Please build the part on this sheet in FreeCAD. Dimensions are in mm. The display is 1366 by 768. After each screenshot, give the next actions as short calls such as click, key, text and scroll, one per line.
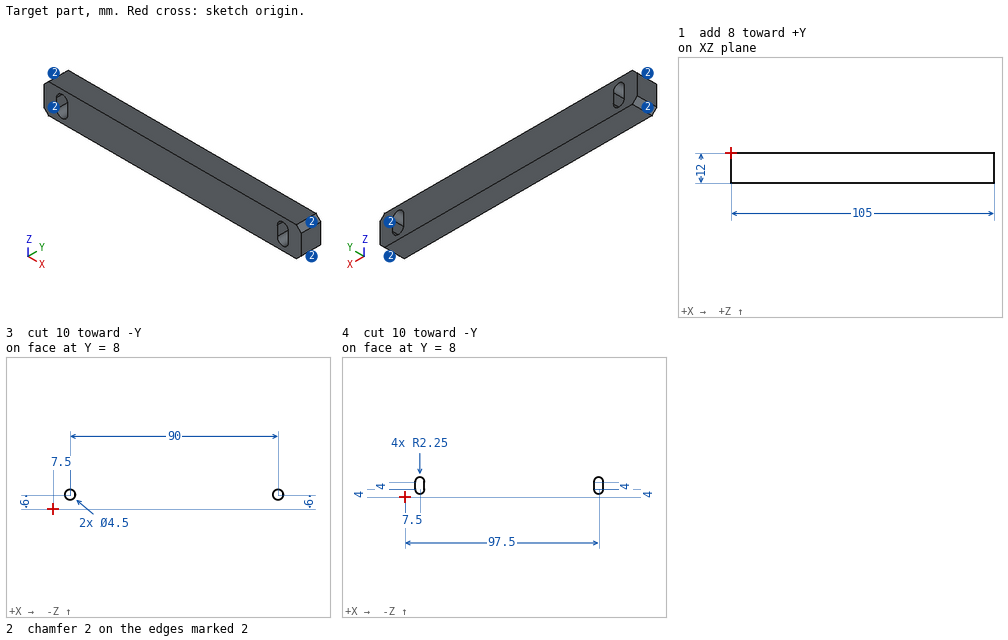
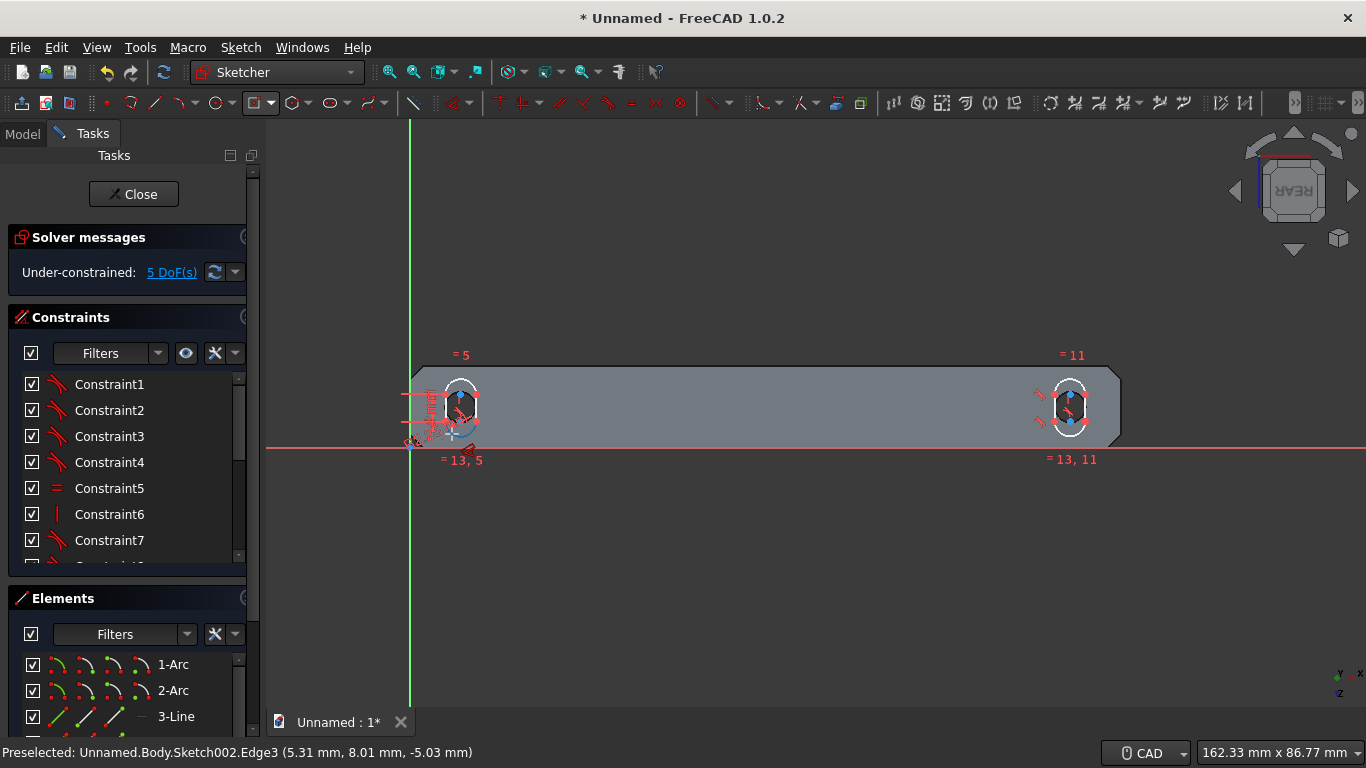
scroll(1055, 413, up, 3)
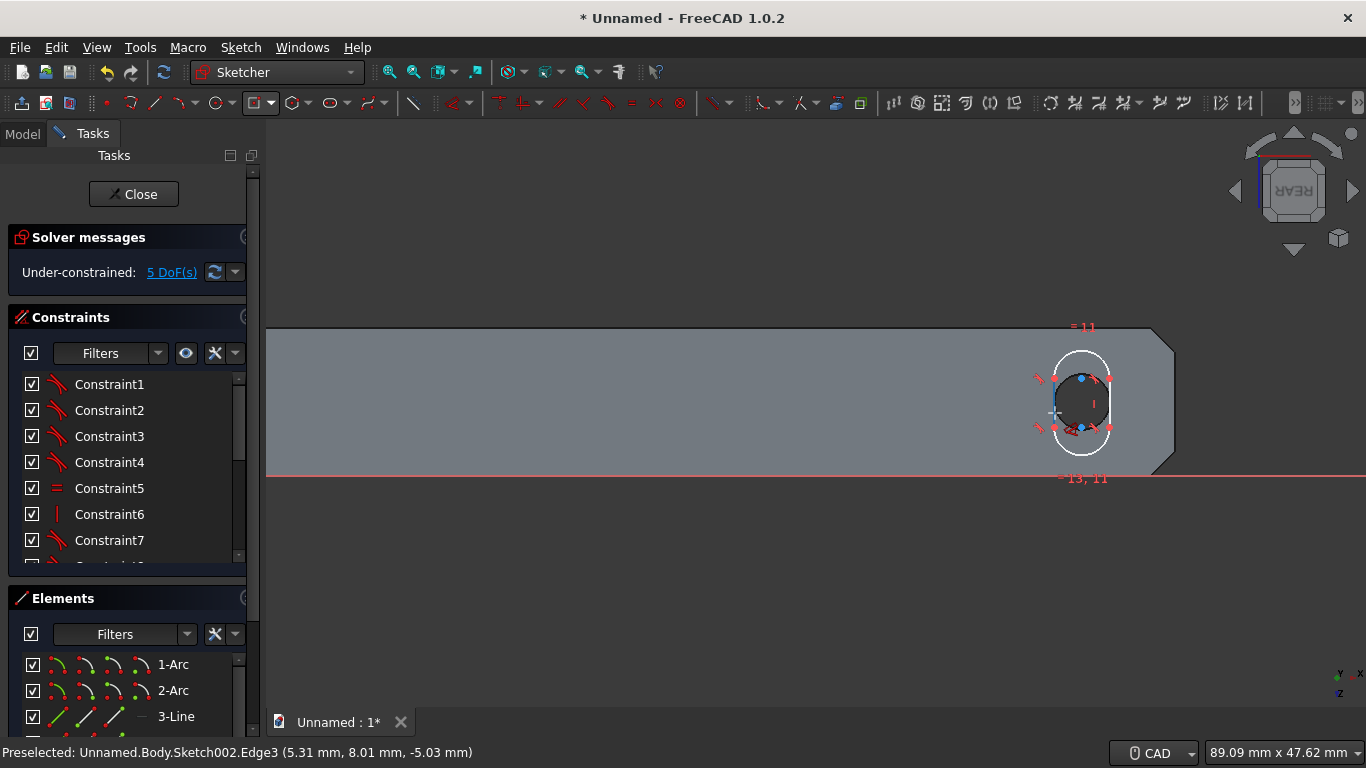
click(1054, 413)
click(1088, 403)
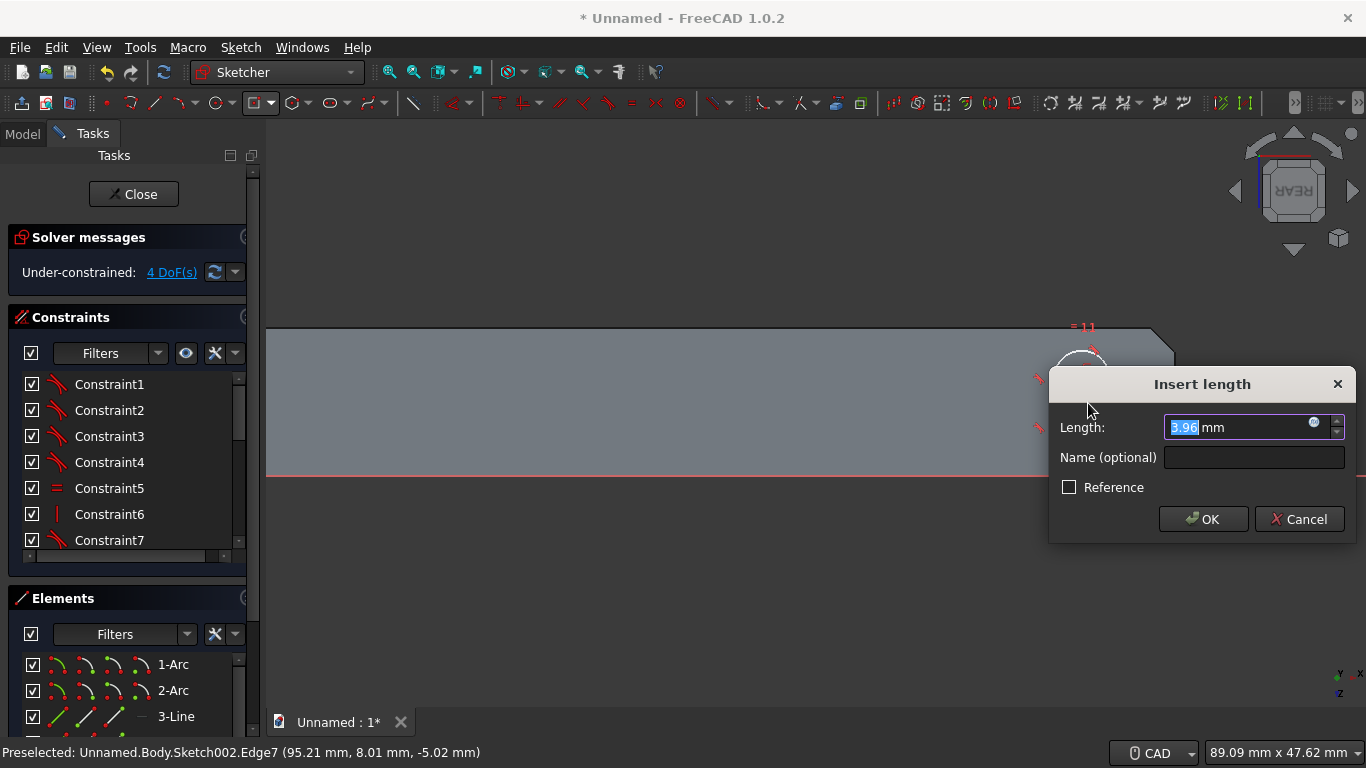
text(4)
key(Return)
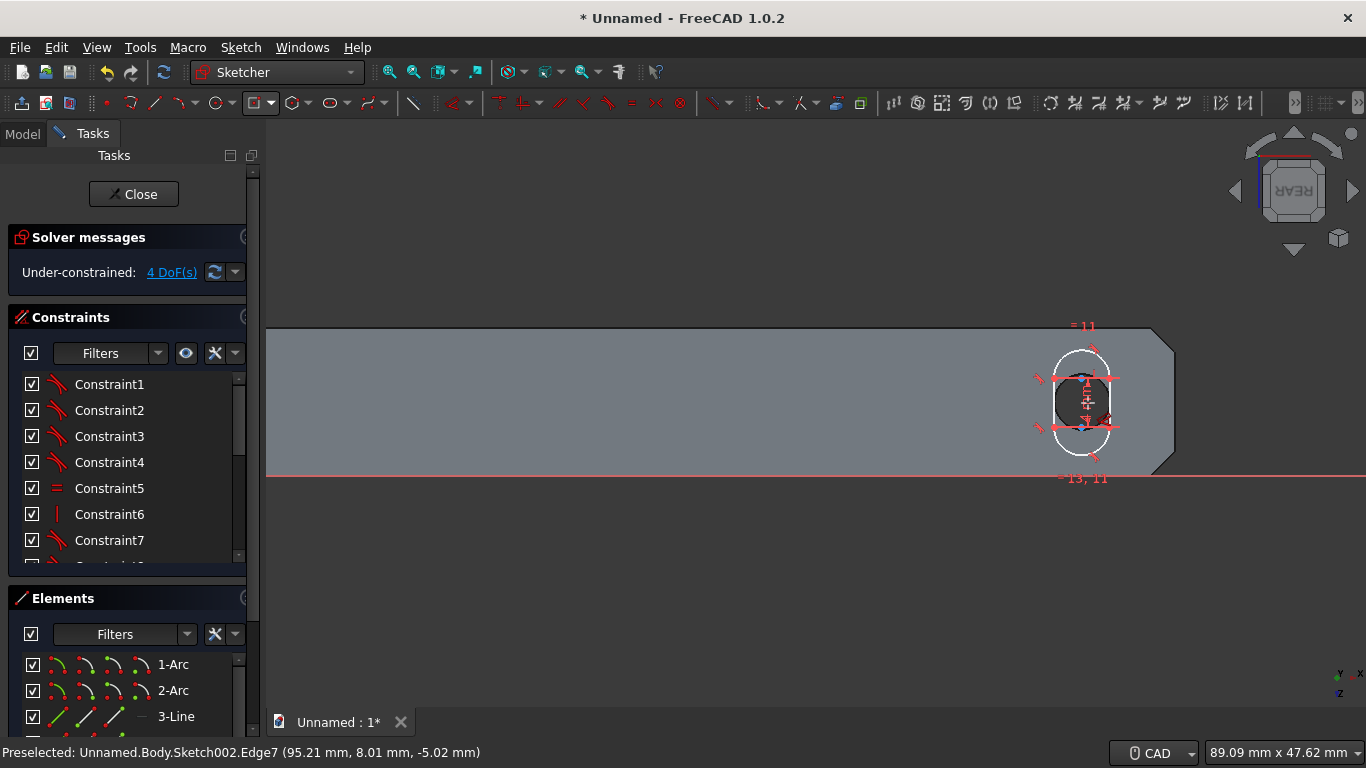
scroll(1056, 413, down, 3)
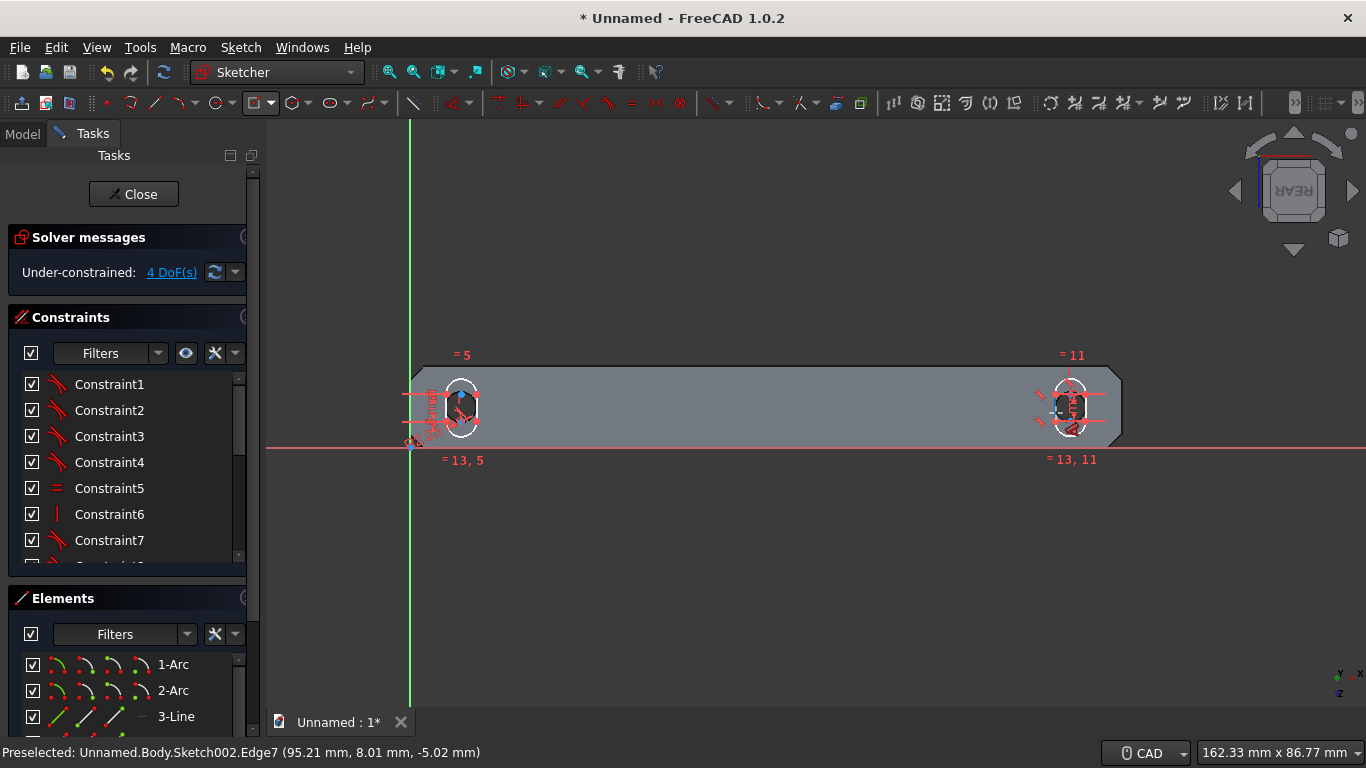
scroll(446, 422, up, 2)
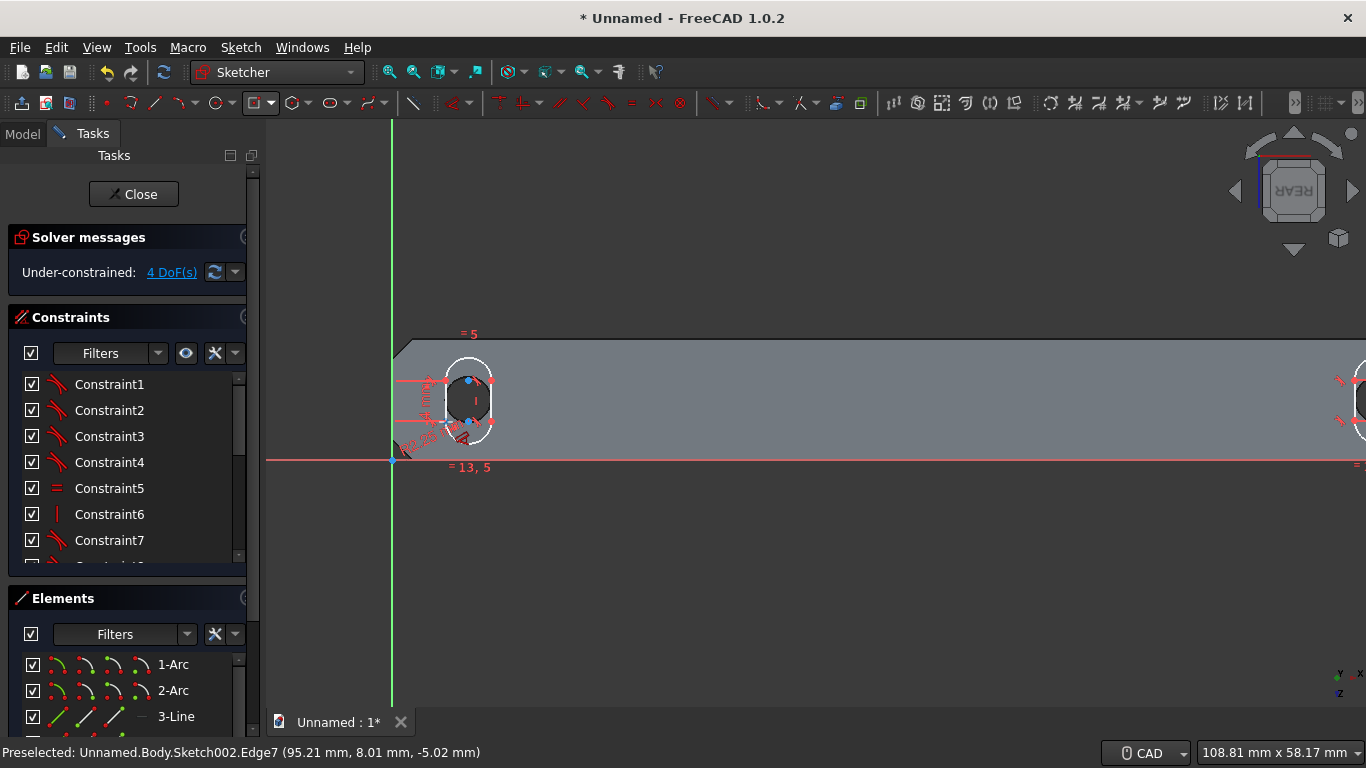
click(446, 421)
click(358, 441)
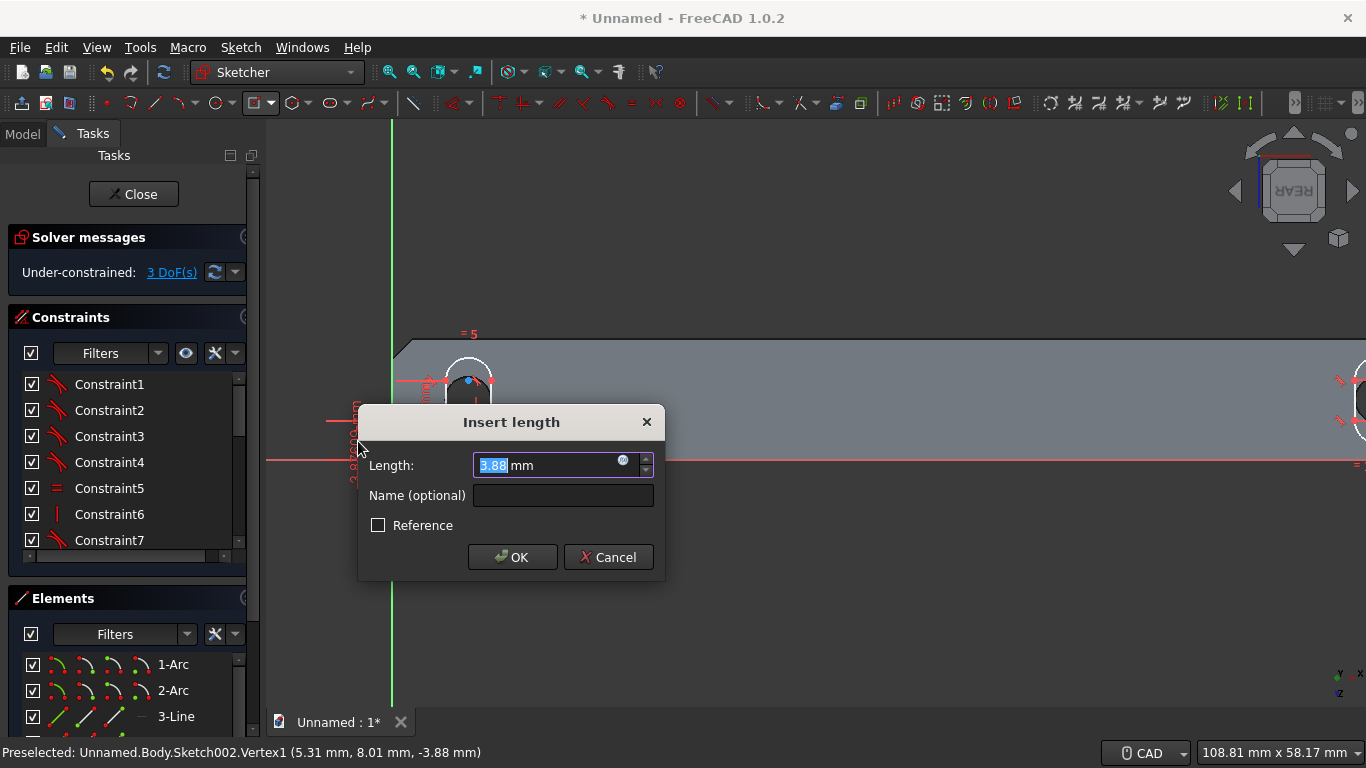
text(4)
key(Return)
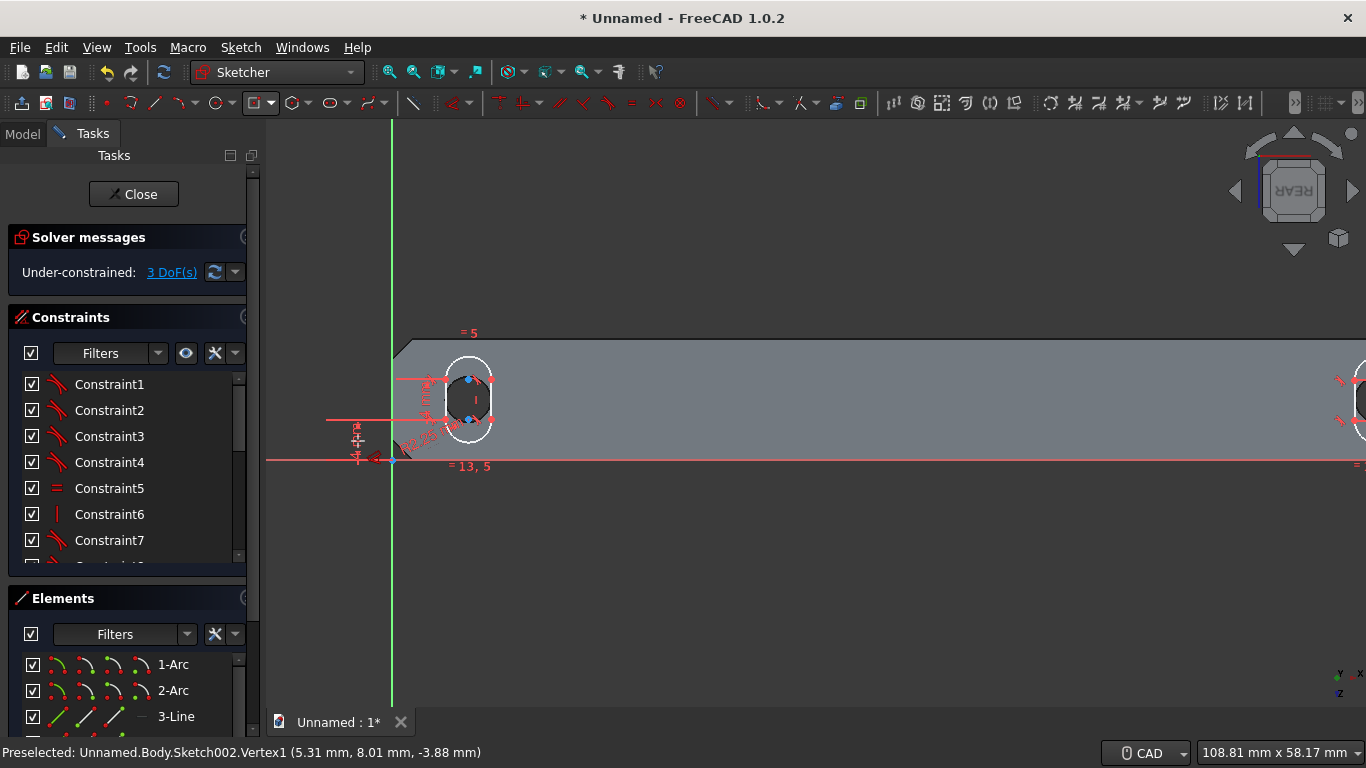
scroll(445, 422, down, 2)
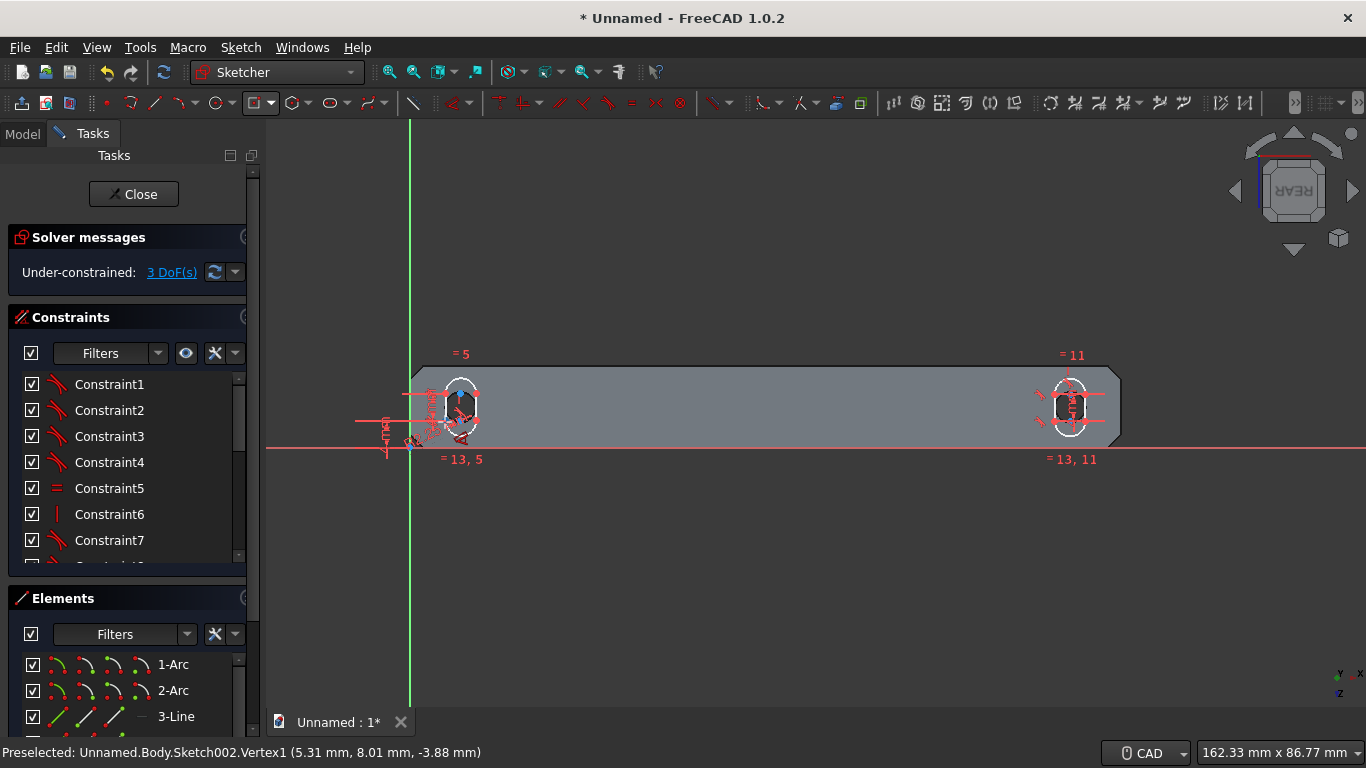
scroll(1055, 421, up, 2)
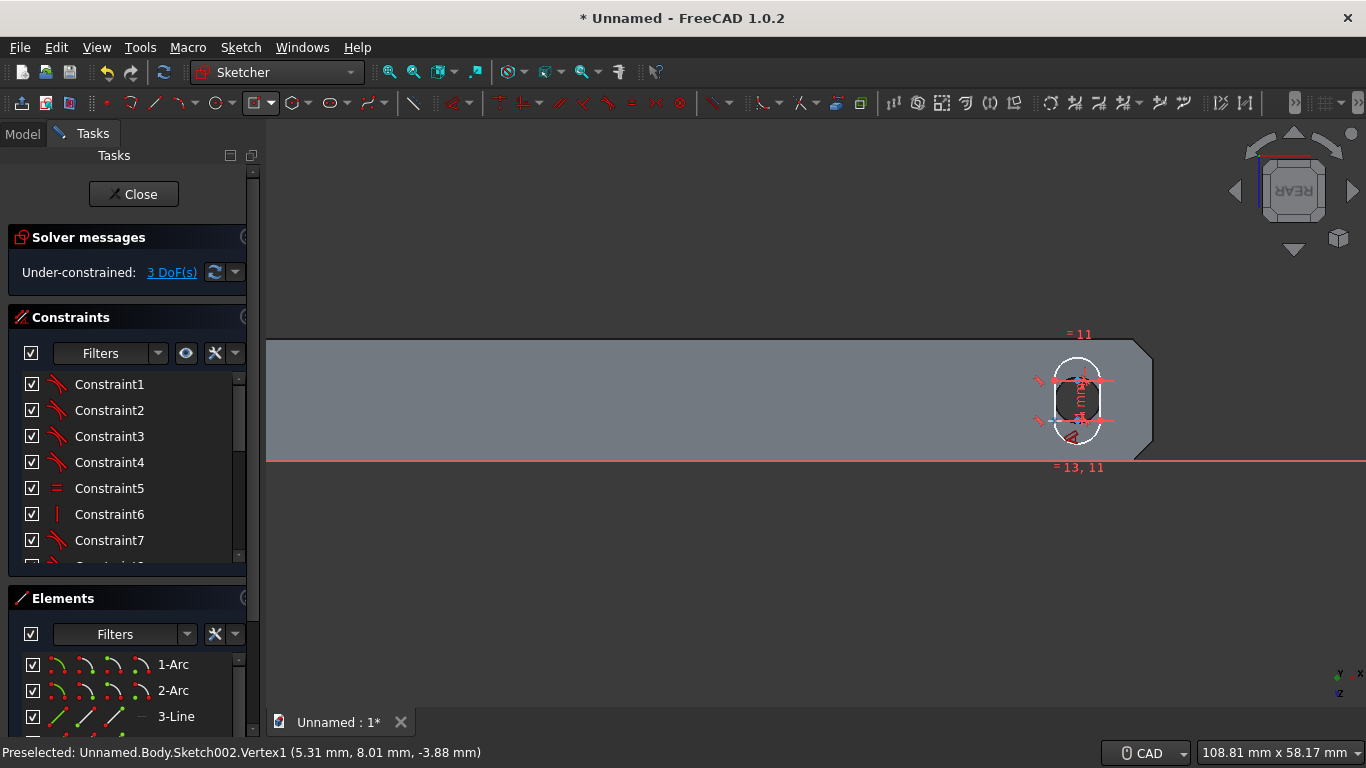
click(1055, 421)
click(1113, 441)